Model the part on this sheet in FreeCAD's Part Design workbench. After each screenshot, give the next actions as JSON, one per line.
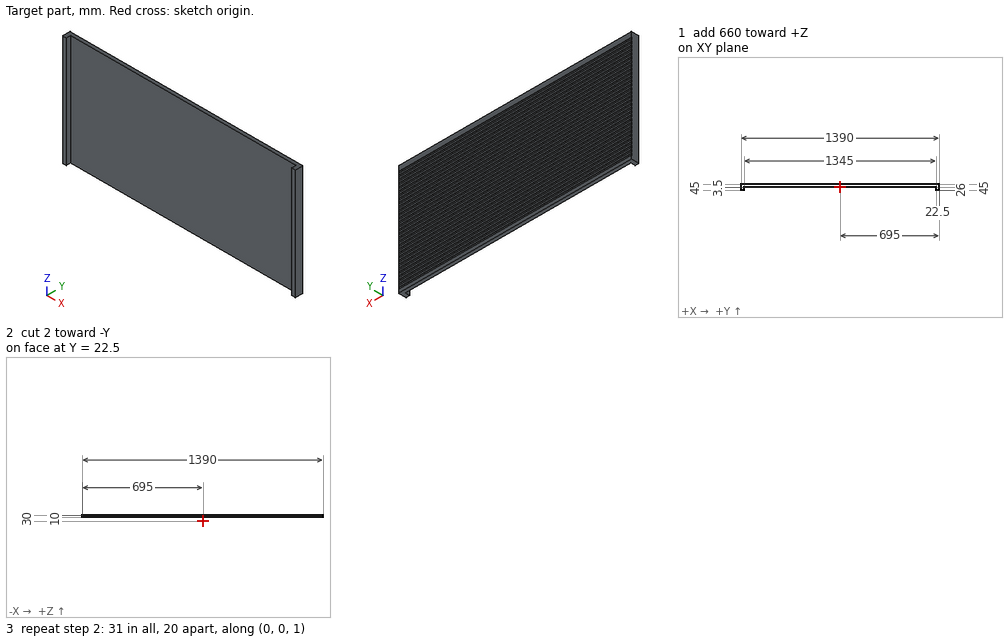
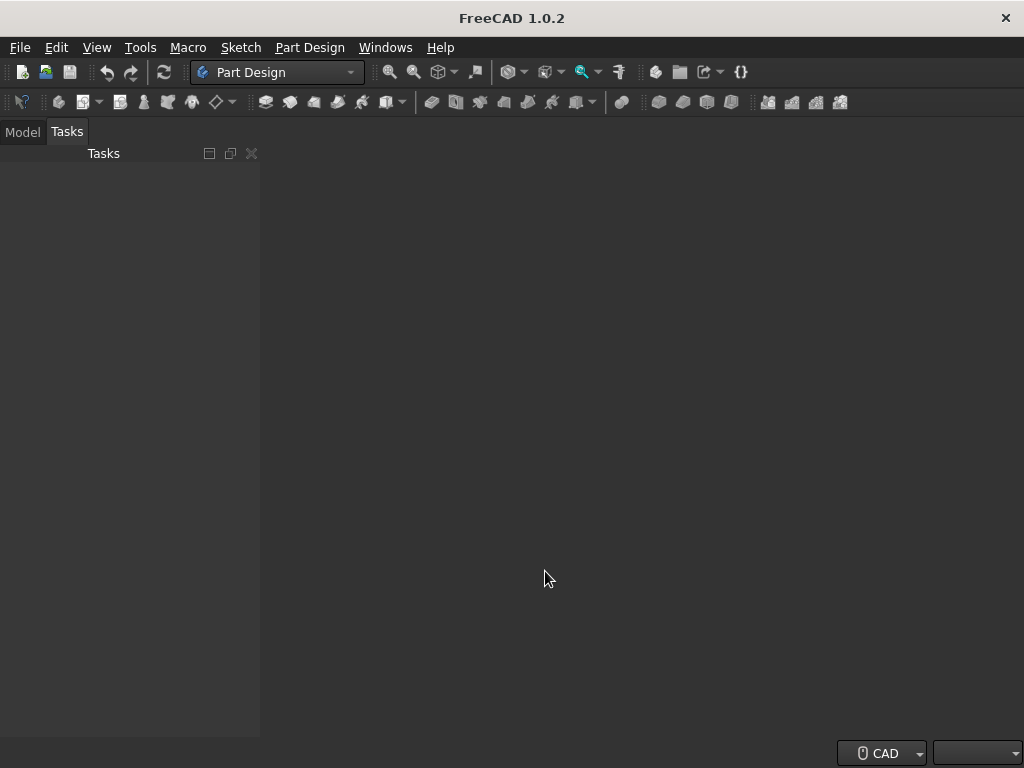
{"action": "key", "text": "ctrl+n"}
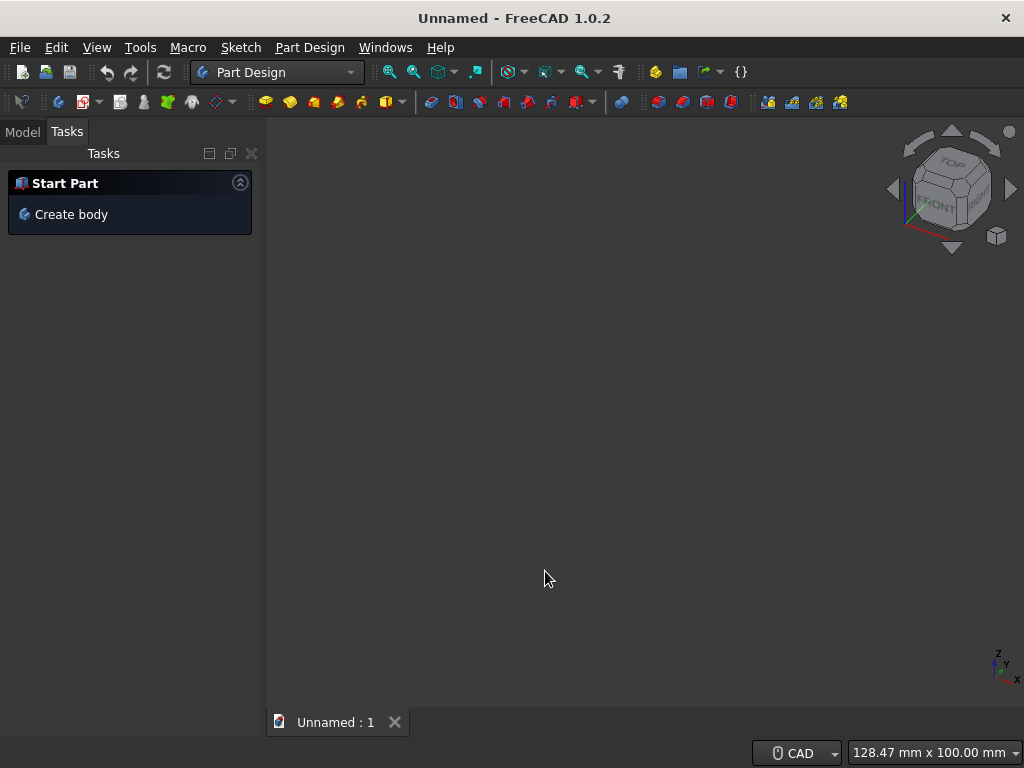
{"action": "left_click", "coordinate": [84, 102]}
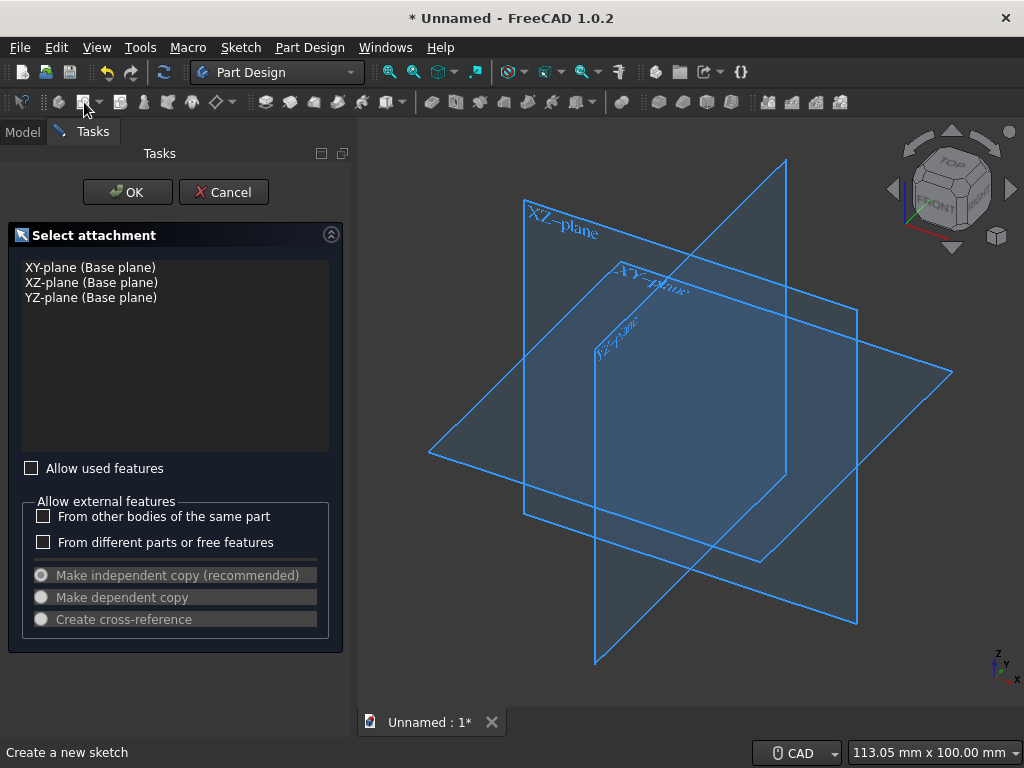
{"action": "left_click", "coordinate": [82, 268]}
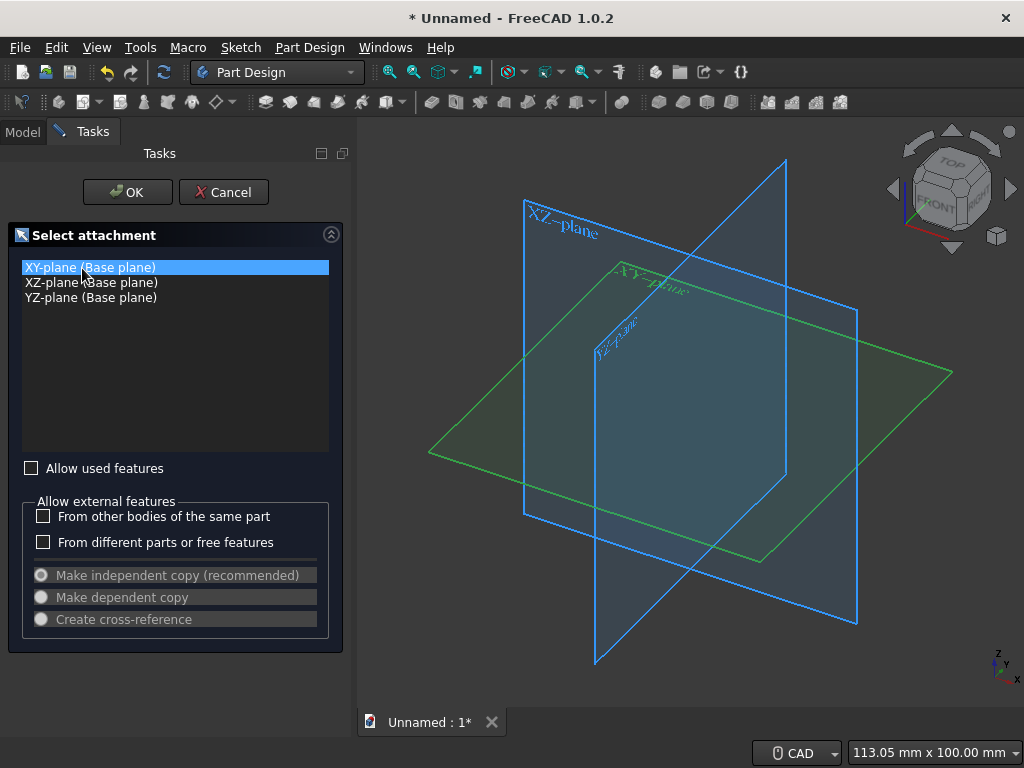
{"action": "left_click", "coordinate": [128, 192]}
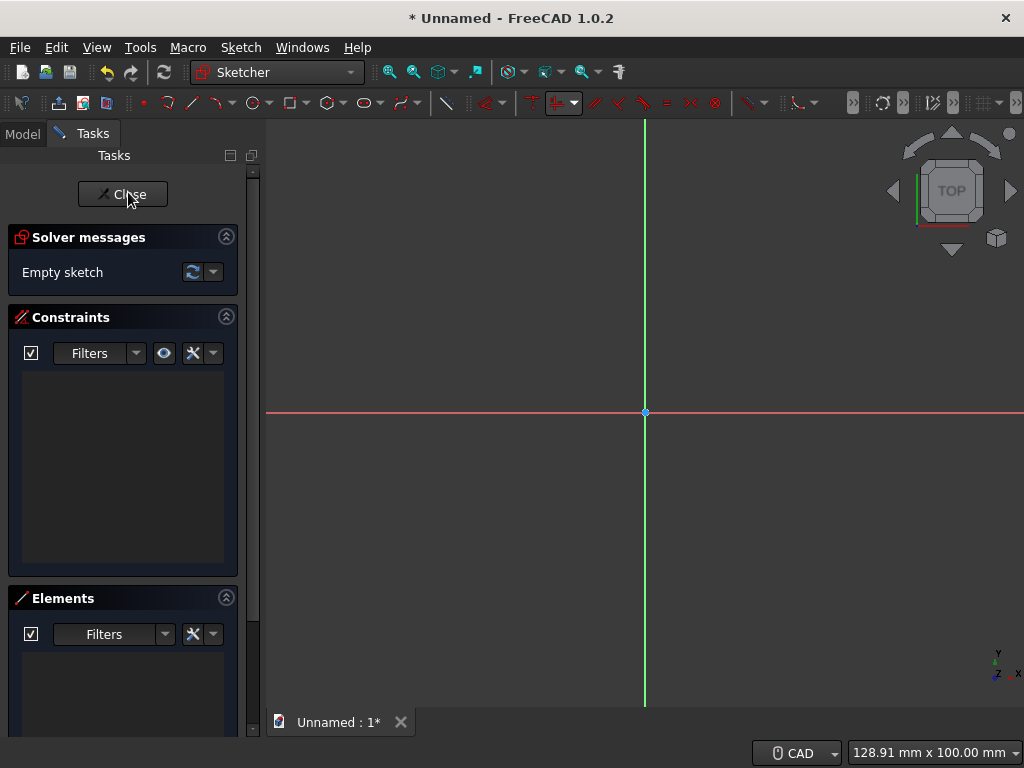
{"action": "scroll", "coordinate": [573, 413], "scroll_direction": "down", "scroll_amount": 15}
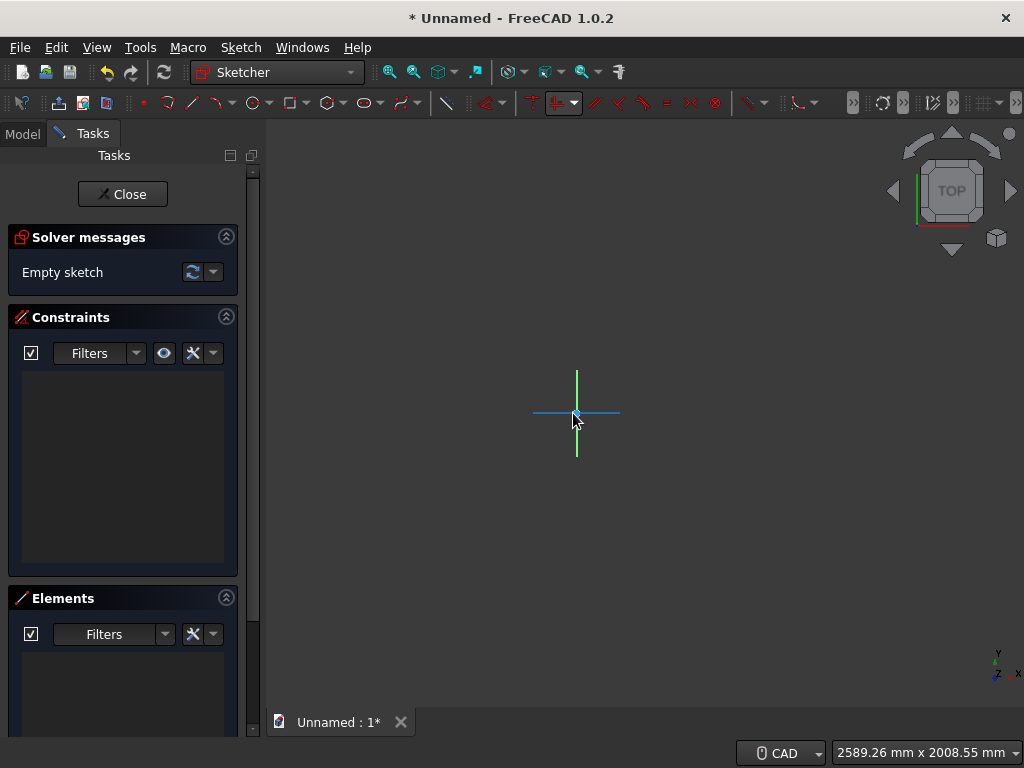
{"action": "left_click", "coordinate": [168, 104]}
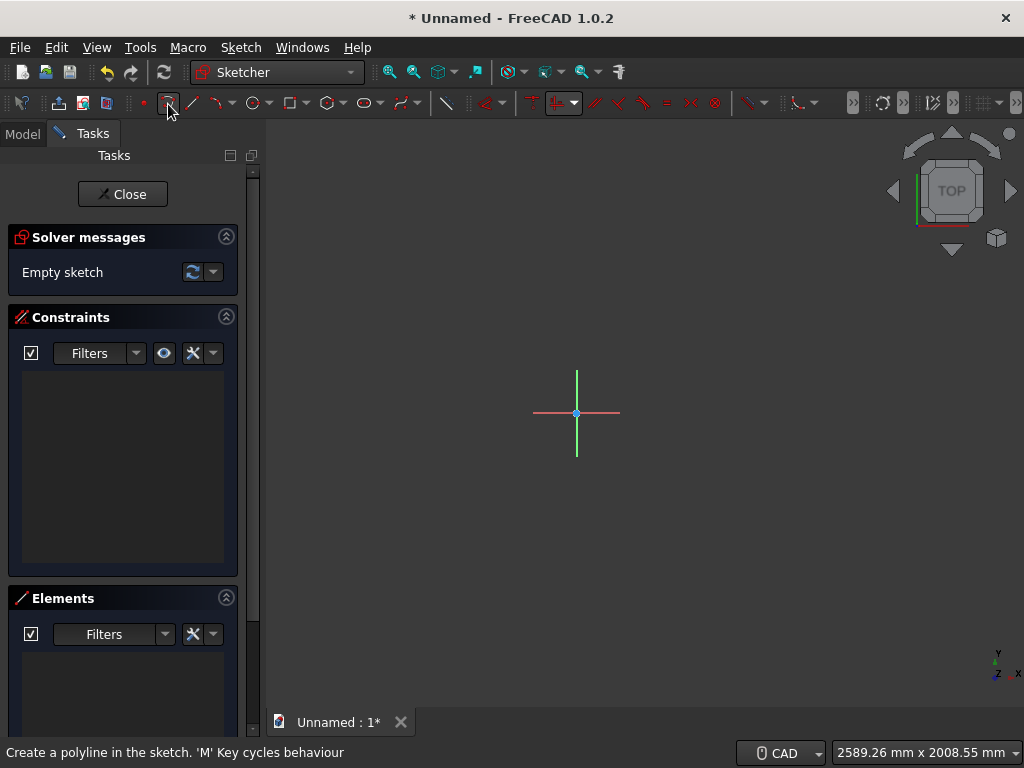
{"action": "scroll", "coordinate": [380, 412], "scroll_direction": "up", "scroll_amount": 14}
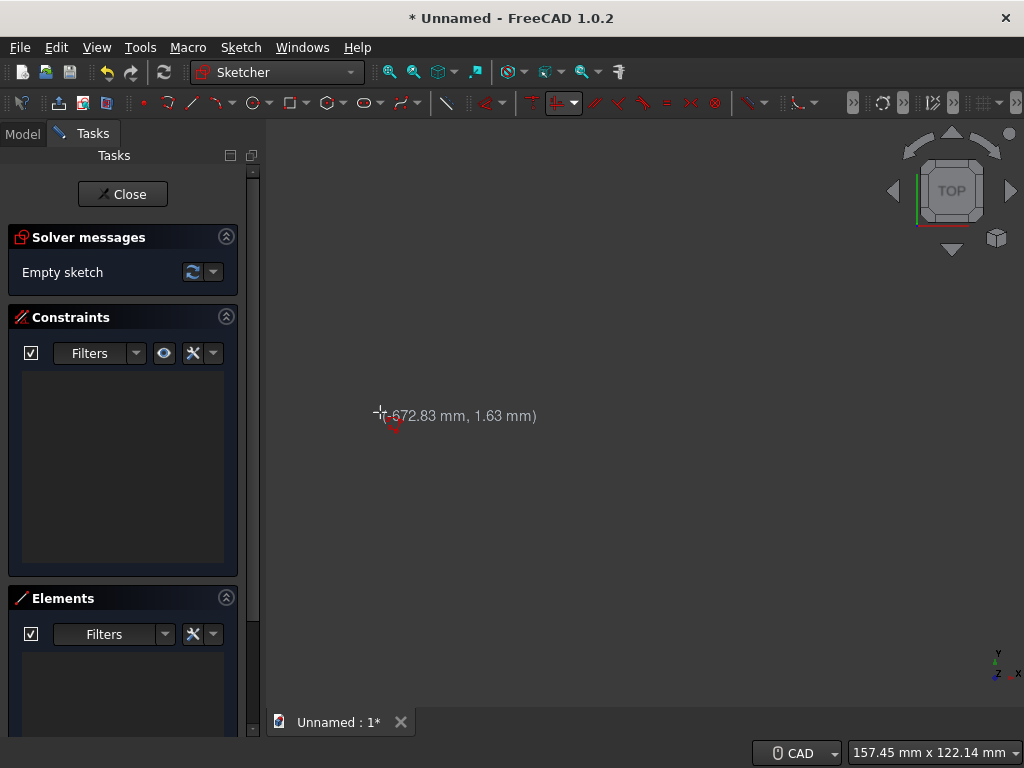
{"action": "left_click", "coordinate": [379, 412]}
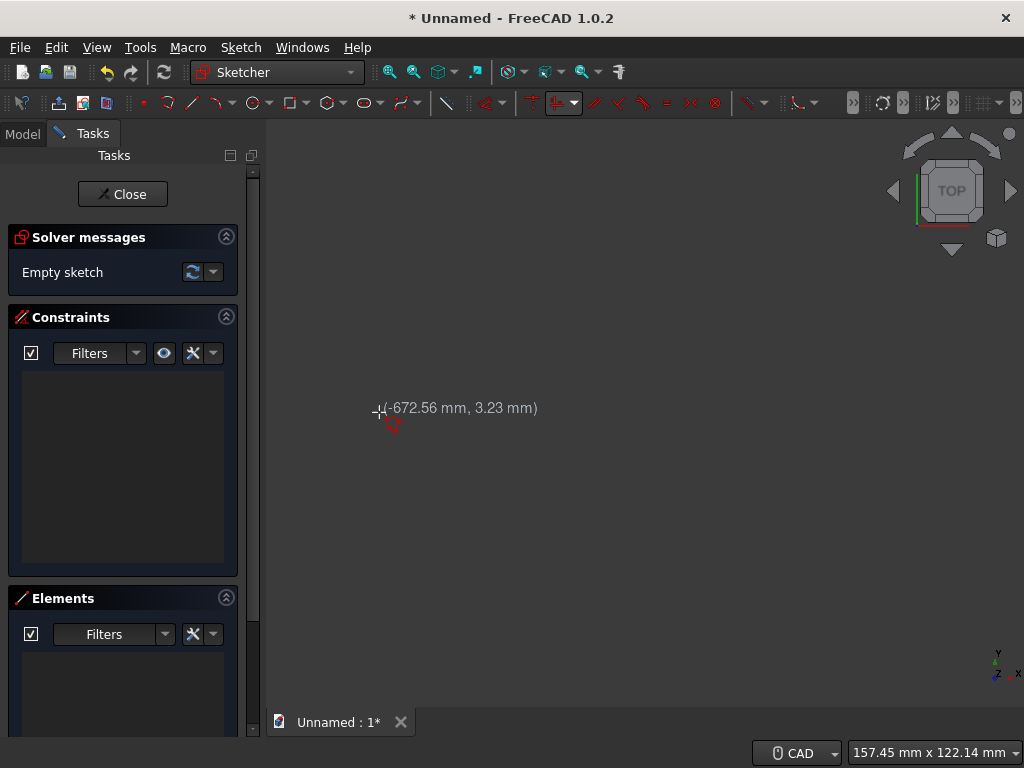
{"action": "scroll", "coordinate": [380, 412], "scroll_direction": "down", "scroll_amount": 14}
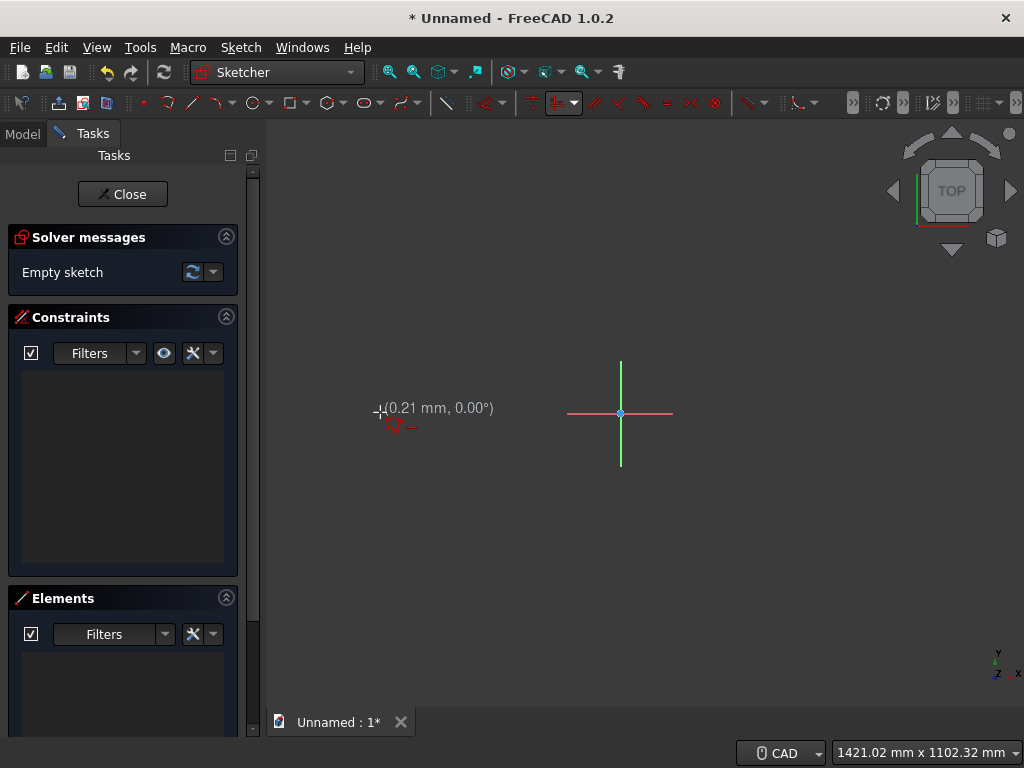
{"action": "scroll", "coordinate": [774, 412], "scroll_direction": "up", "scroll_amount": 14}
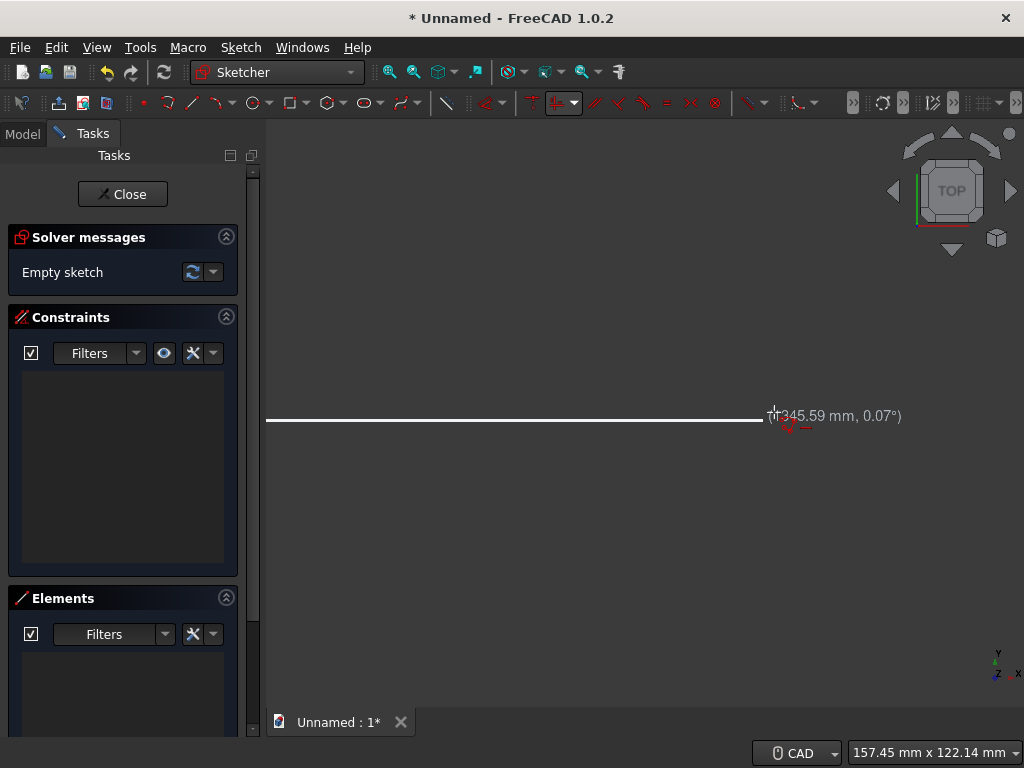
{"action": "left_click", "coordinate": [761, 412]}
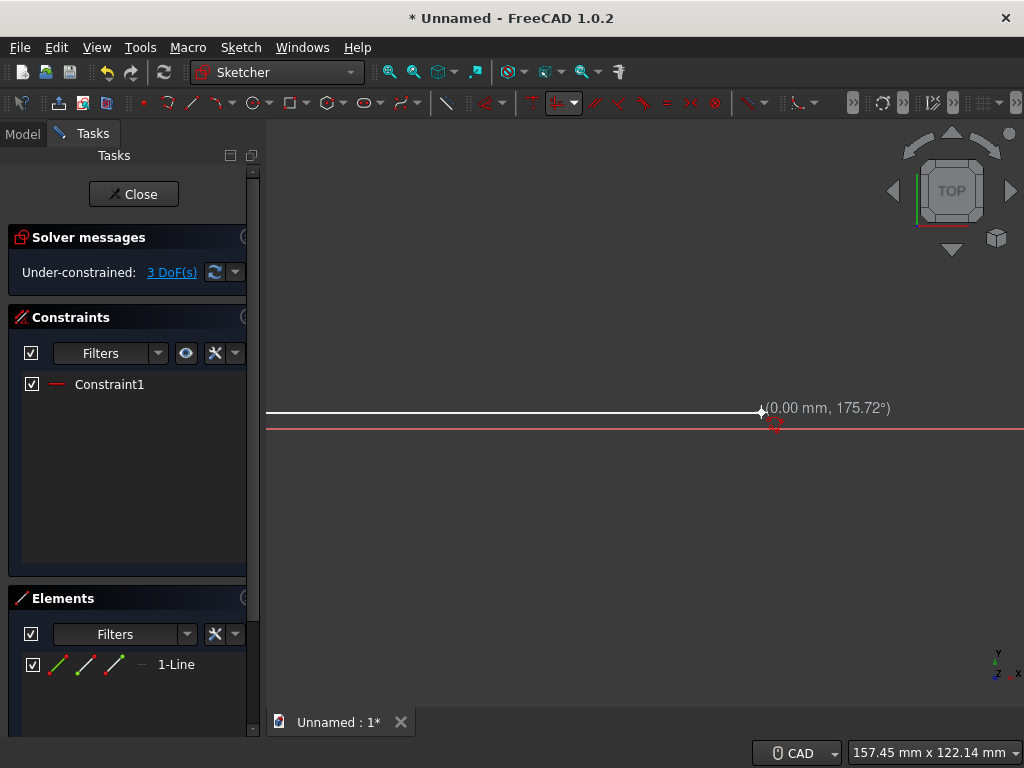
{"action": "scroll", "coordinate": [774, 412], "scroll_direction": "down", "scroll_amount": 14}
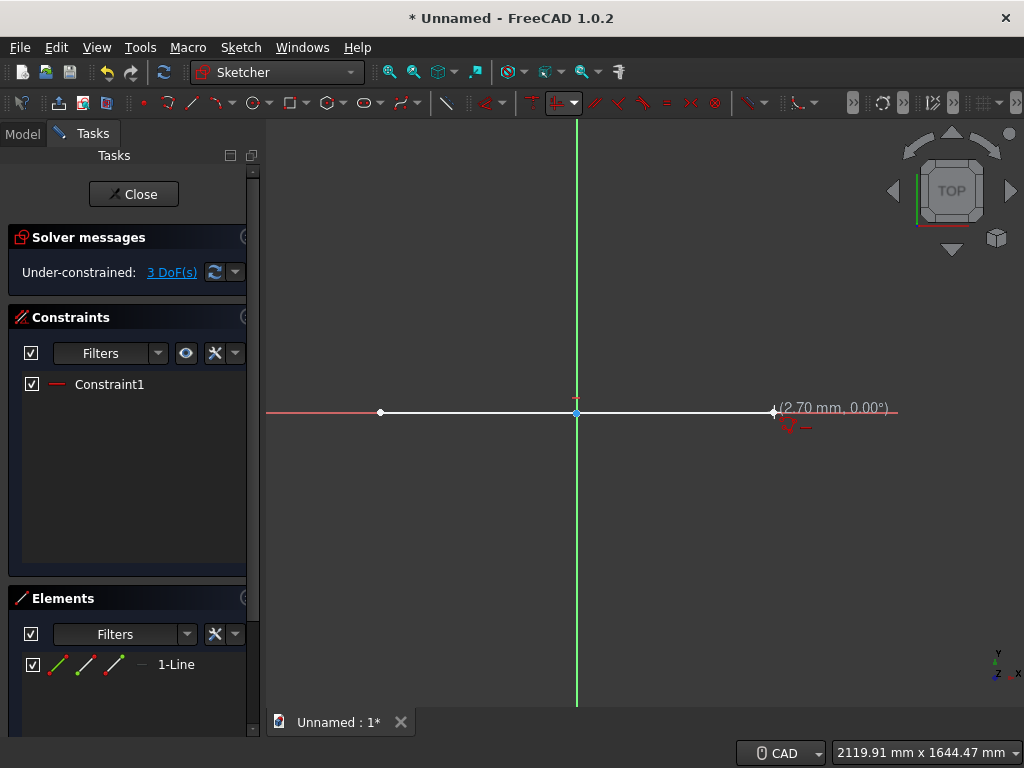
{"action": "scroll", "coordinate": [774, 420], "scroll_direction": "up", "scroll_amount": 5}